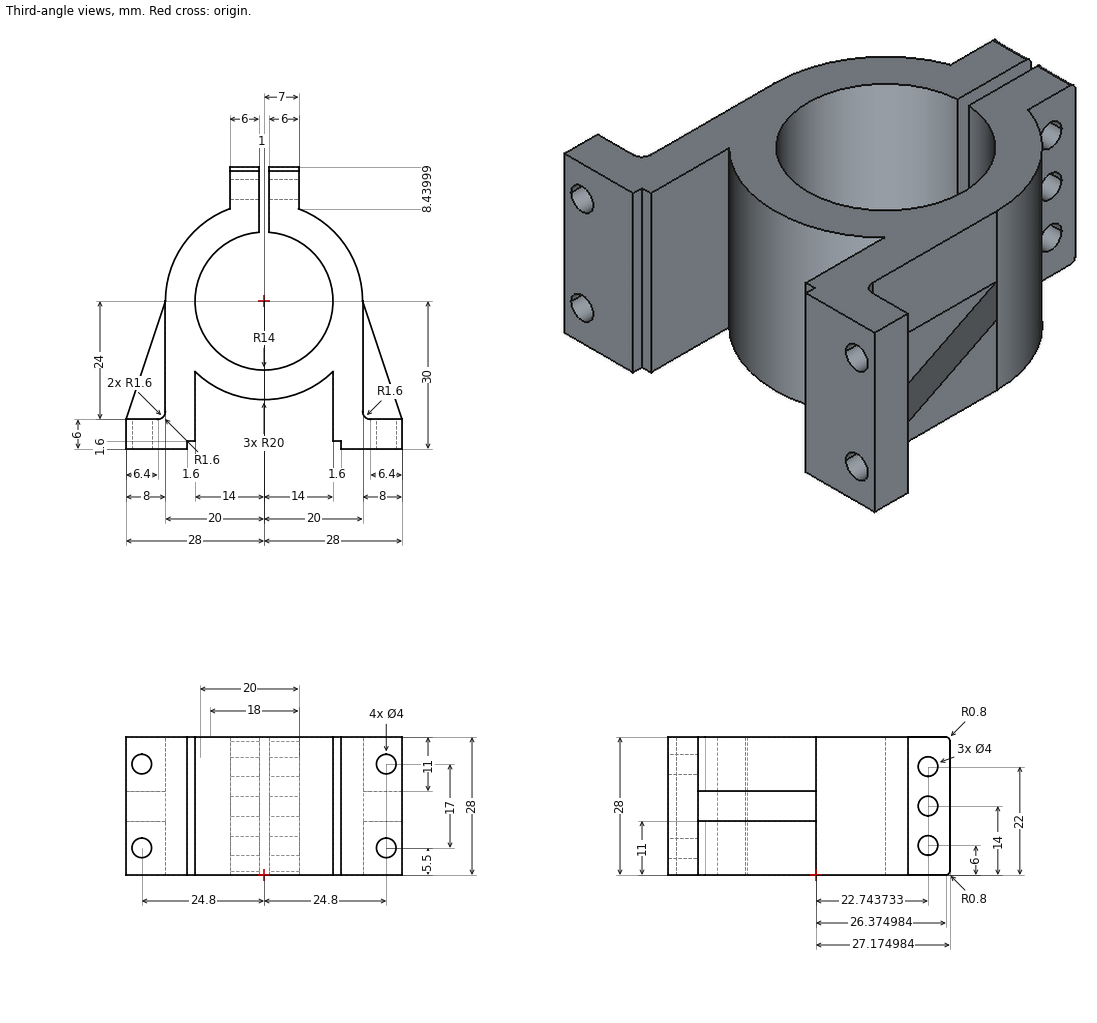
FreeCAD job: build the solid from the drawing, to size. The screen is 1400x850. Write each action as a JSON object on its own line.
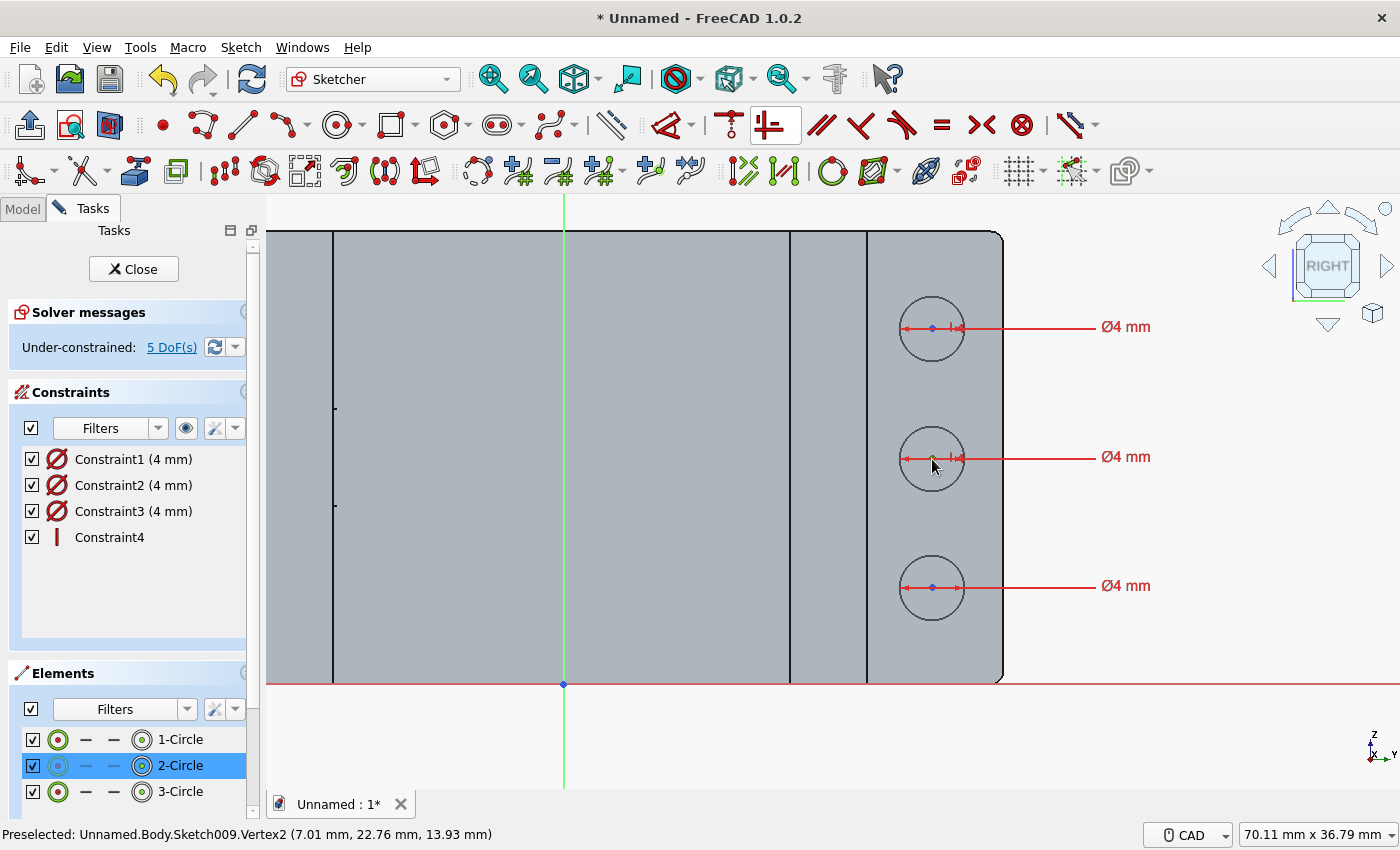
{"action": "left_click", "coordinate": [932, 588]}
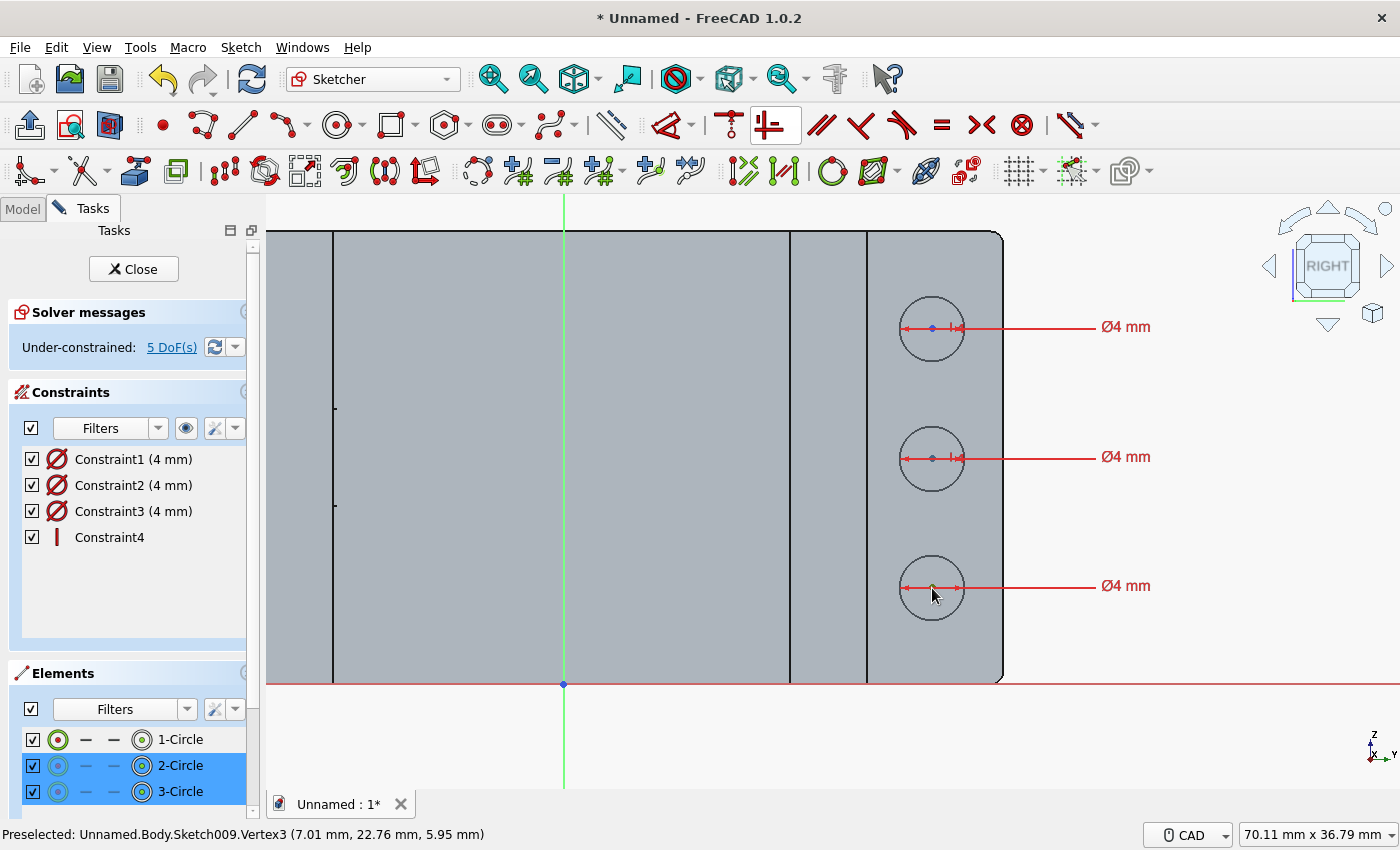
{"action": "left_click", "coordinate": [796, 126]}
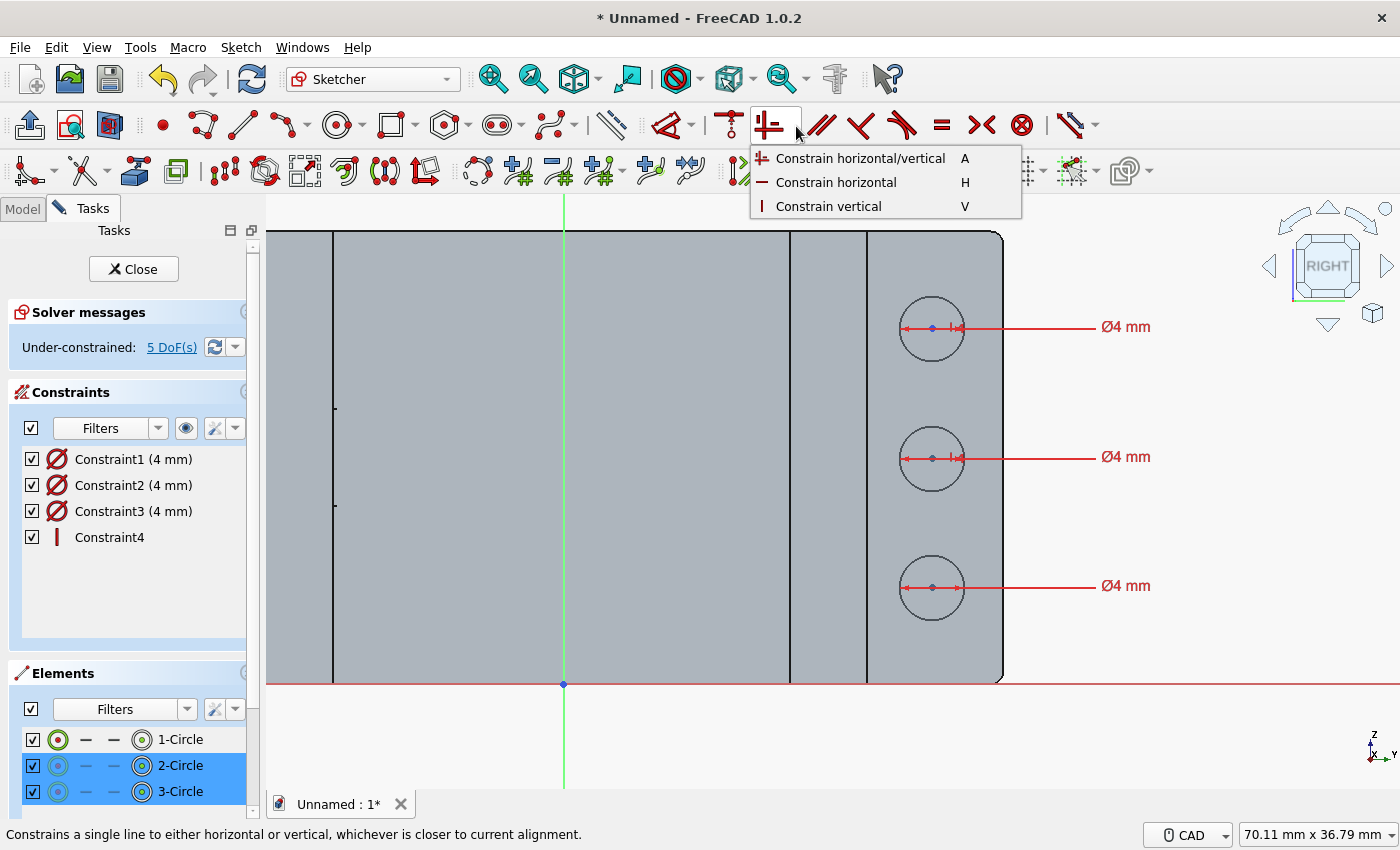
{"action": "left_click", "coordinate": [886, 206]}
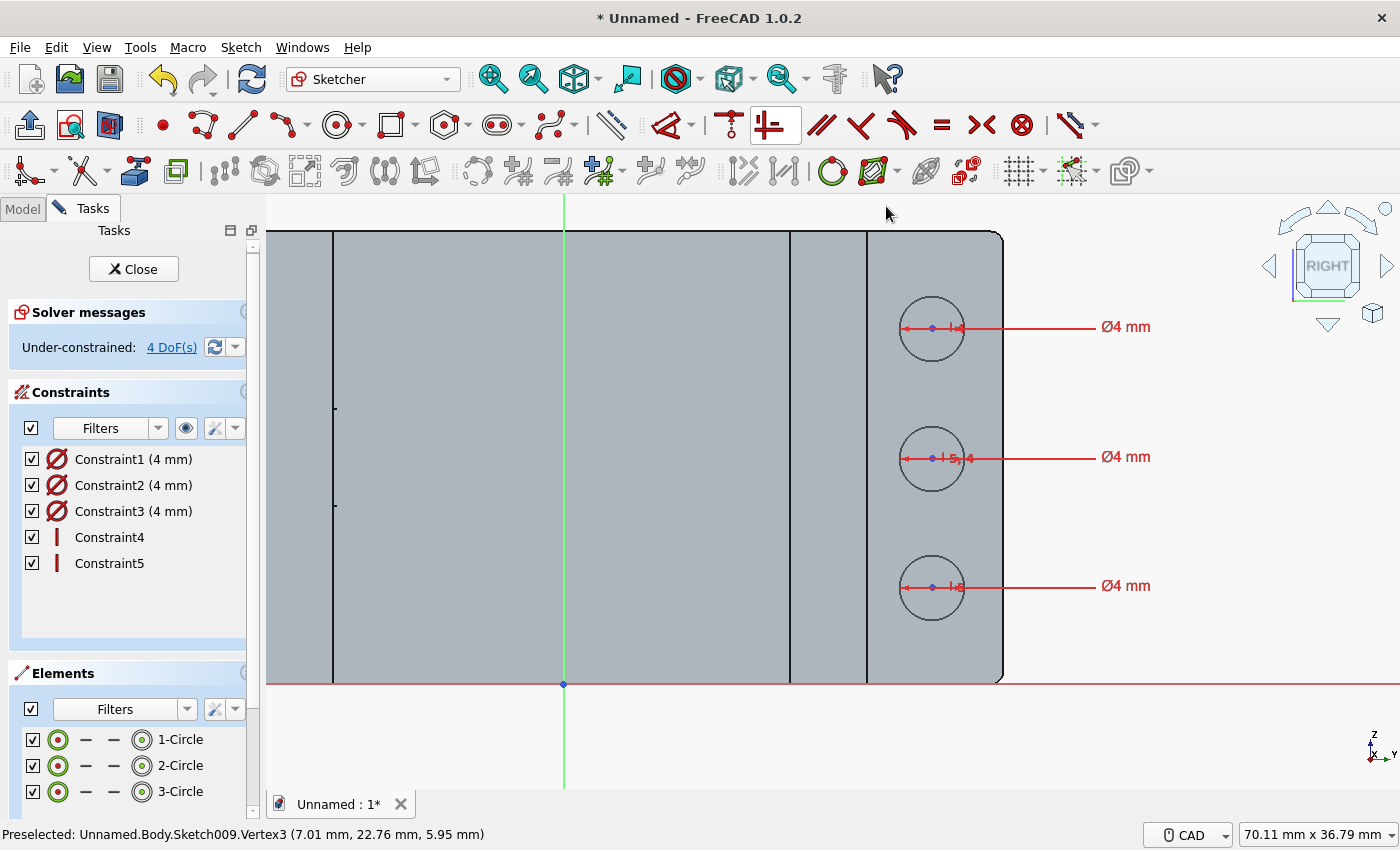
{"action": "left_click", "coordinate": [666, 126]}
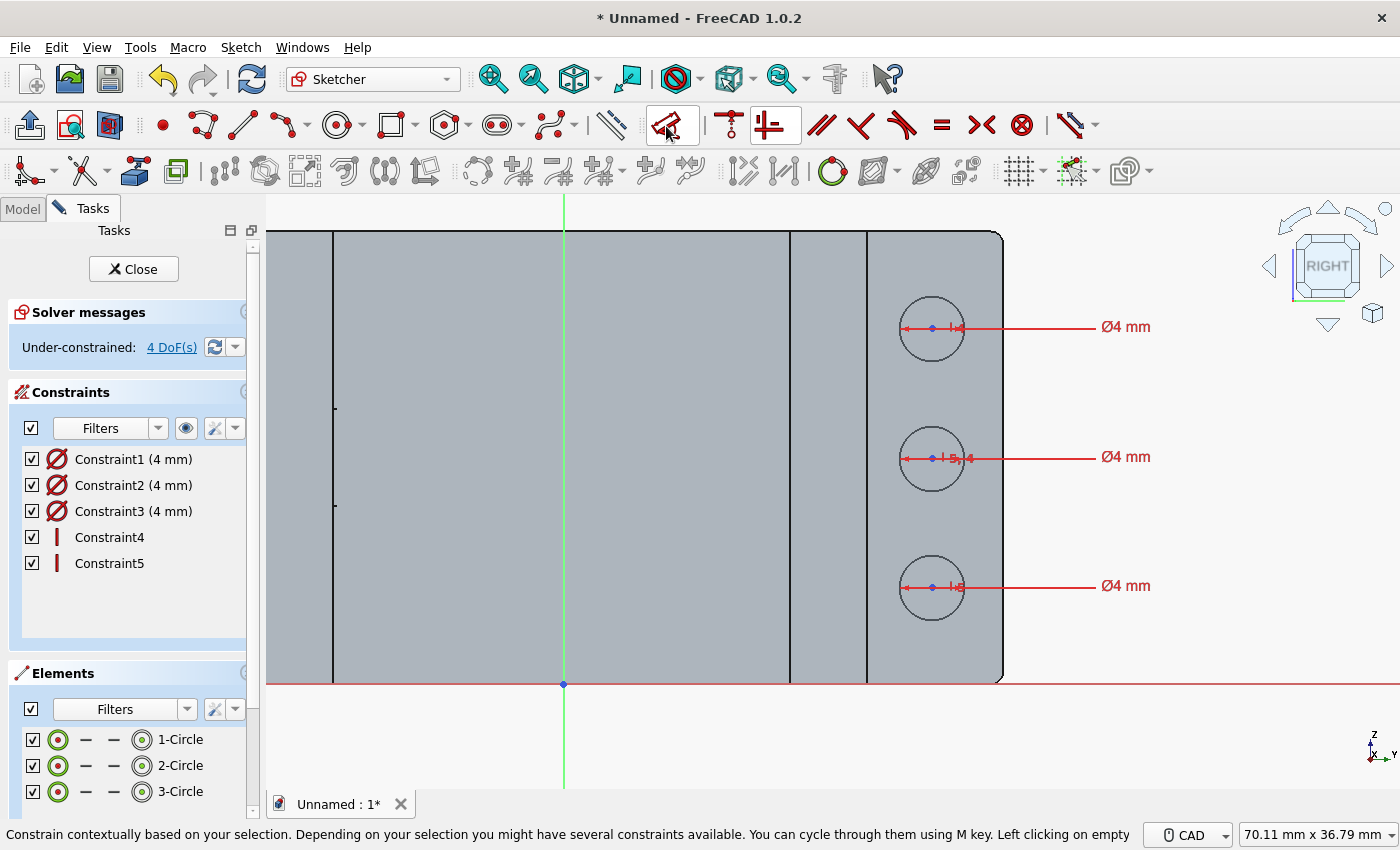
{"action": "left_click", "coordinate": [932, 588]}
{"action": "left_click", "coordinate": [530, 636]}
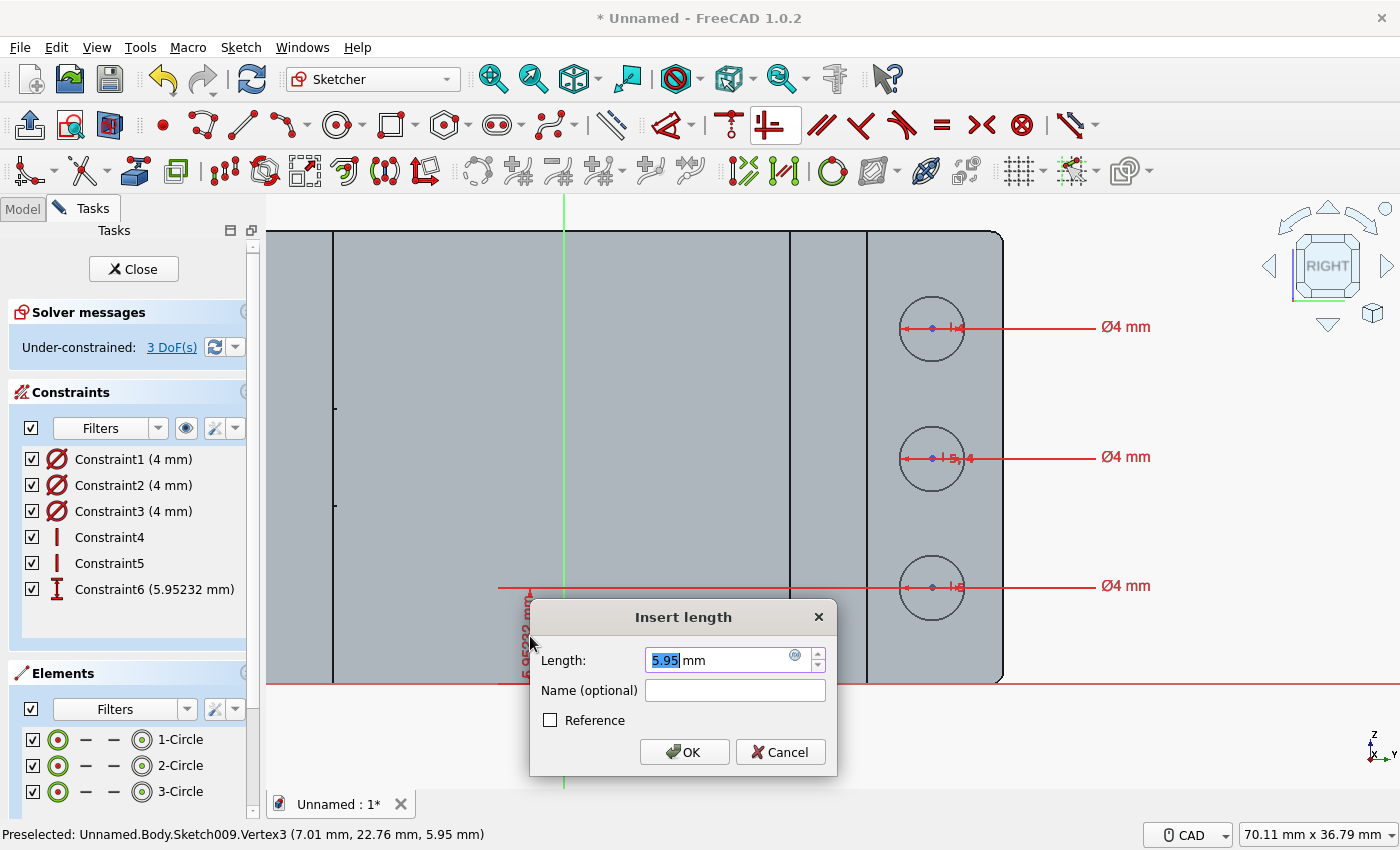
{"action": "type", "text": "6"}
{"action": "key", "text": "Return"}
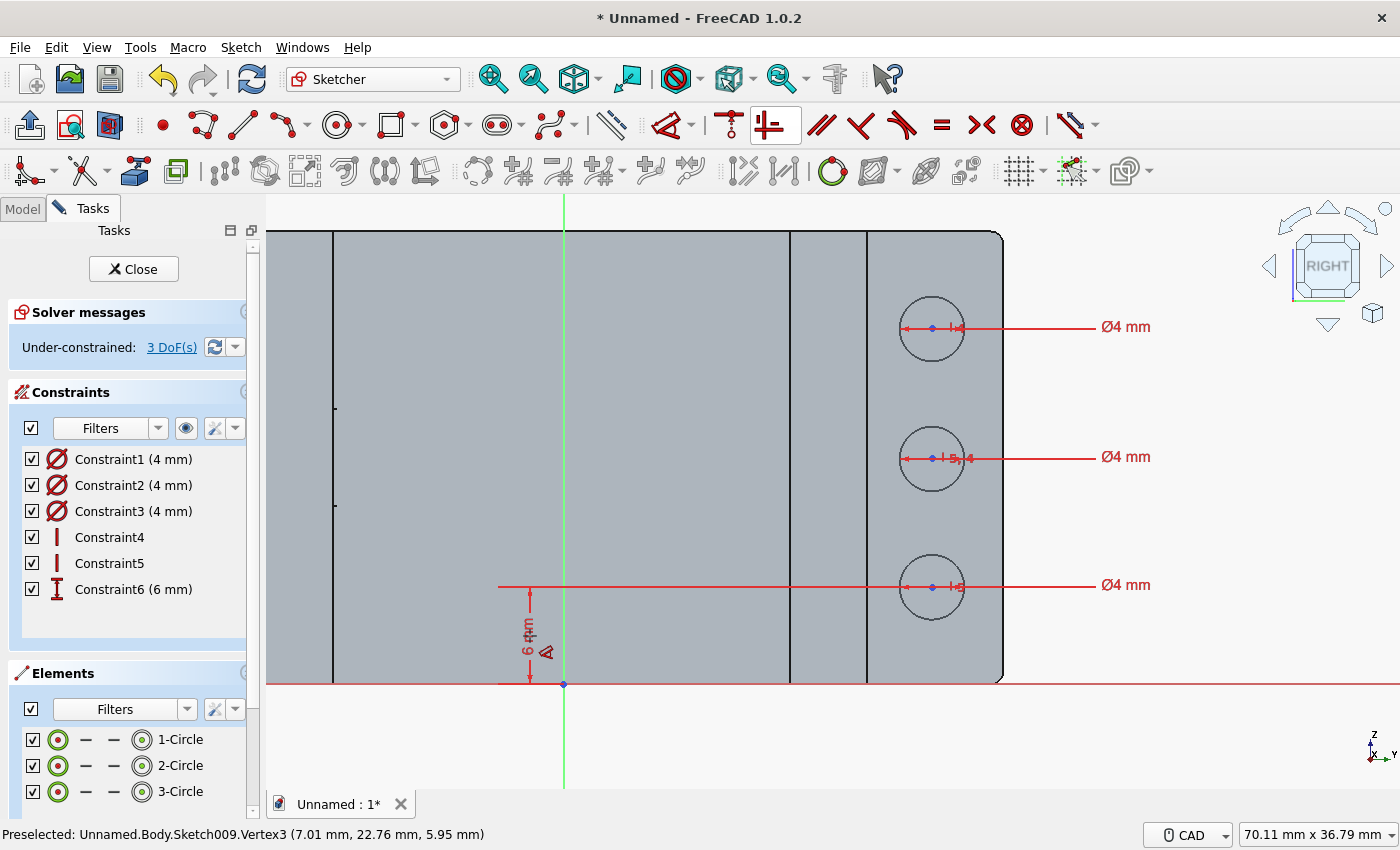
{"action": "left_click", "coordinate": [932, 329]}
{"action": "left_click", "coordinate": [530, 507]}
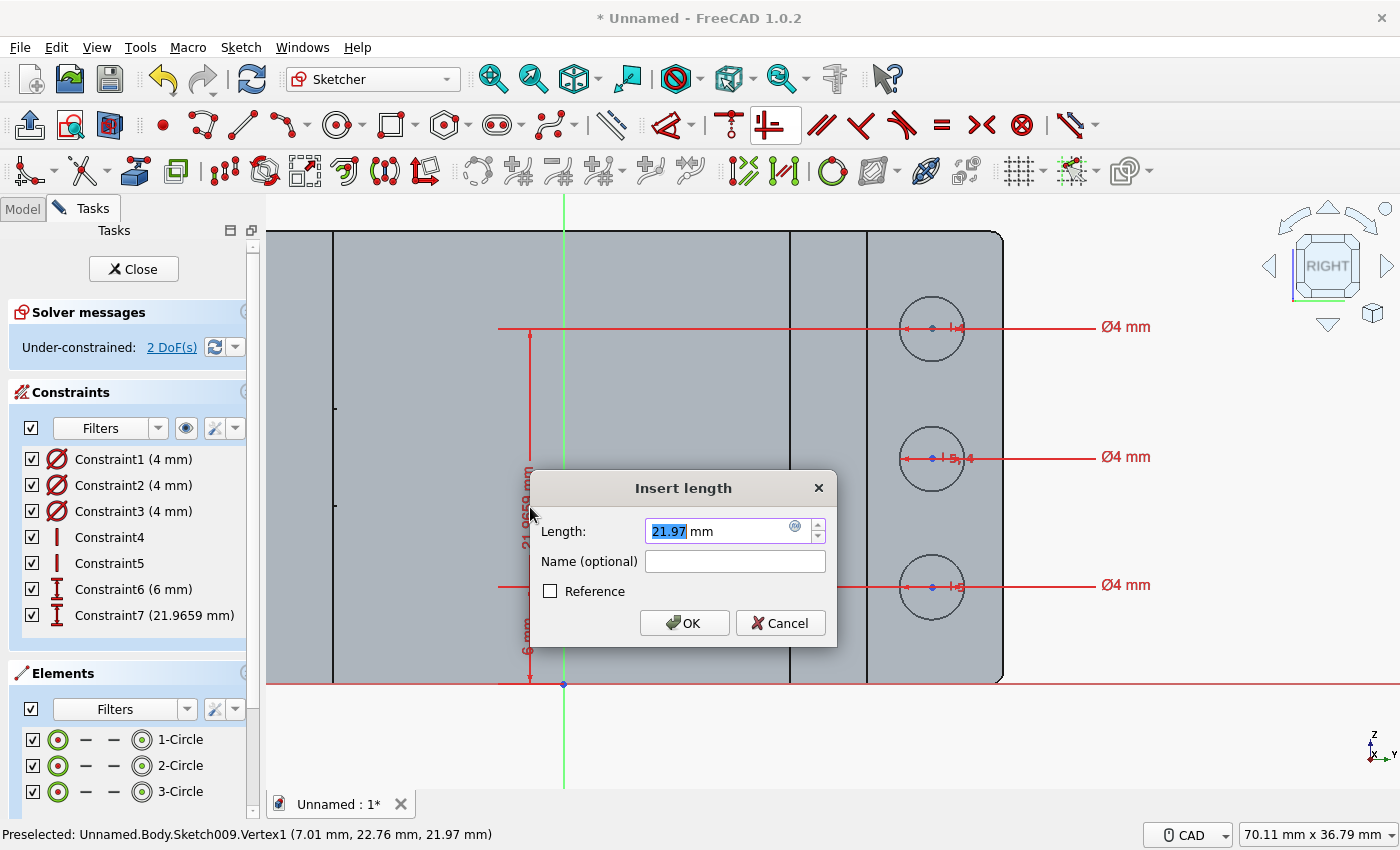
{"action": "type", "text": "22"}
{"action": "key", "text": "Return"}